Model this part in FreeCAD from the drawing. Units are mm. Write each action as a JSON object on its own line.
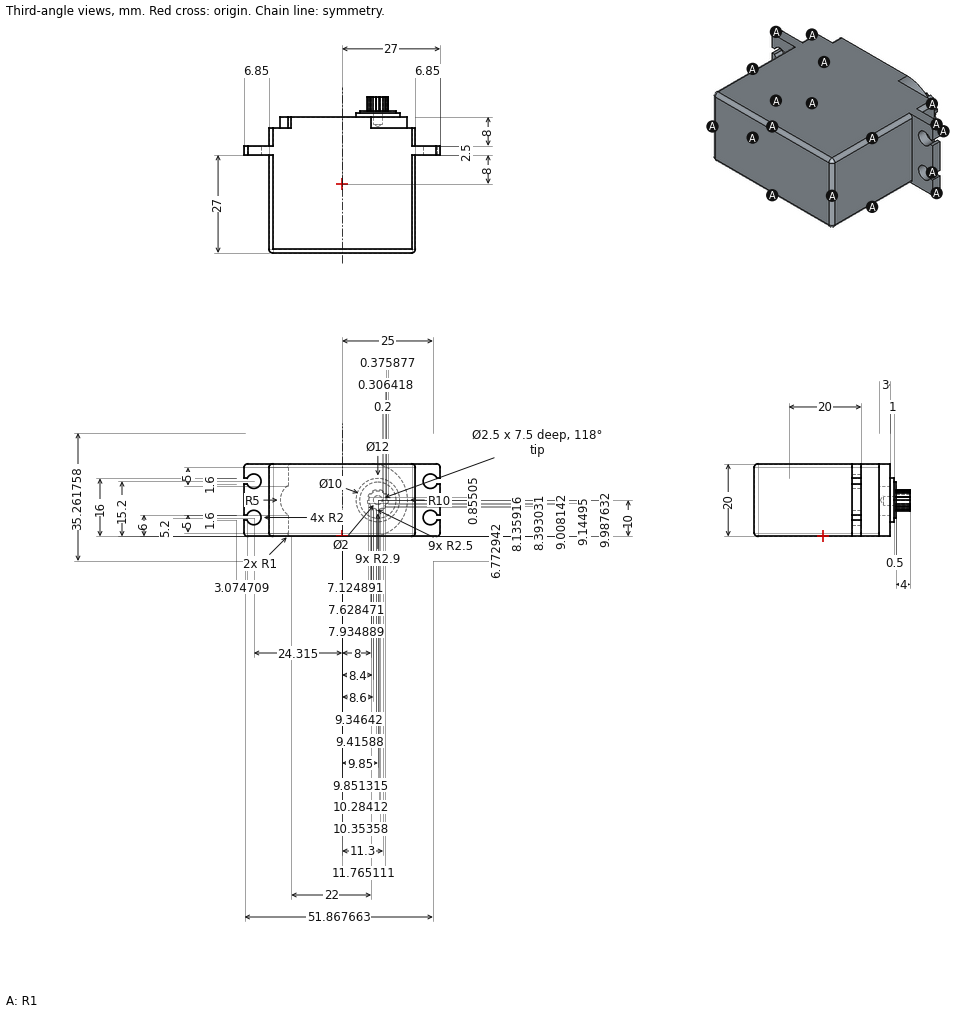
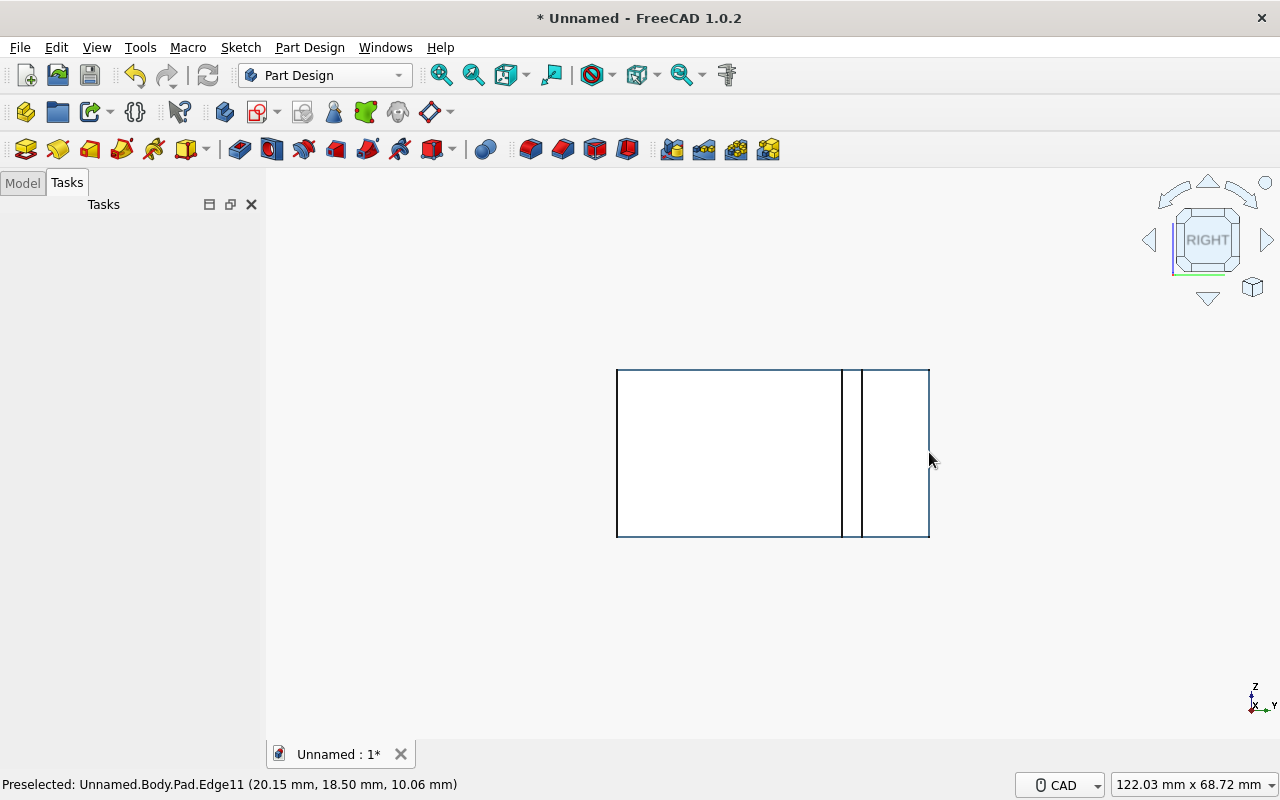
{"action": "key", "text": "5"}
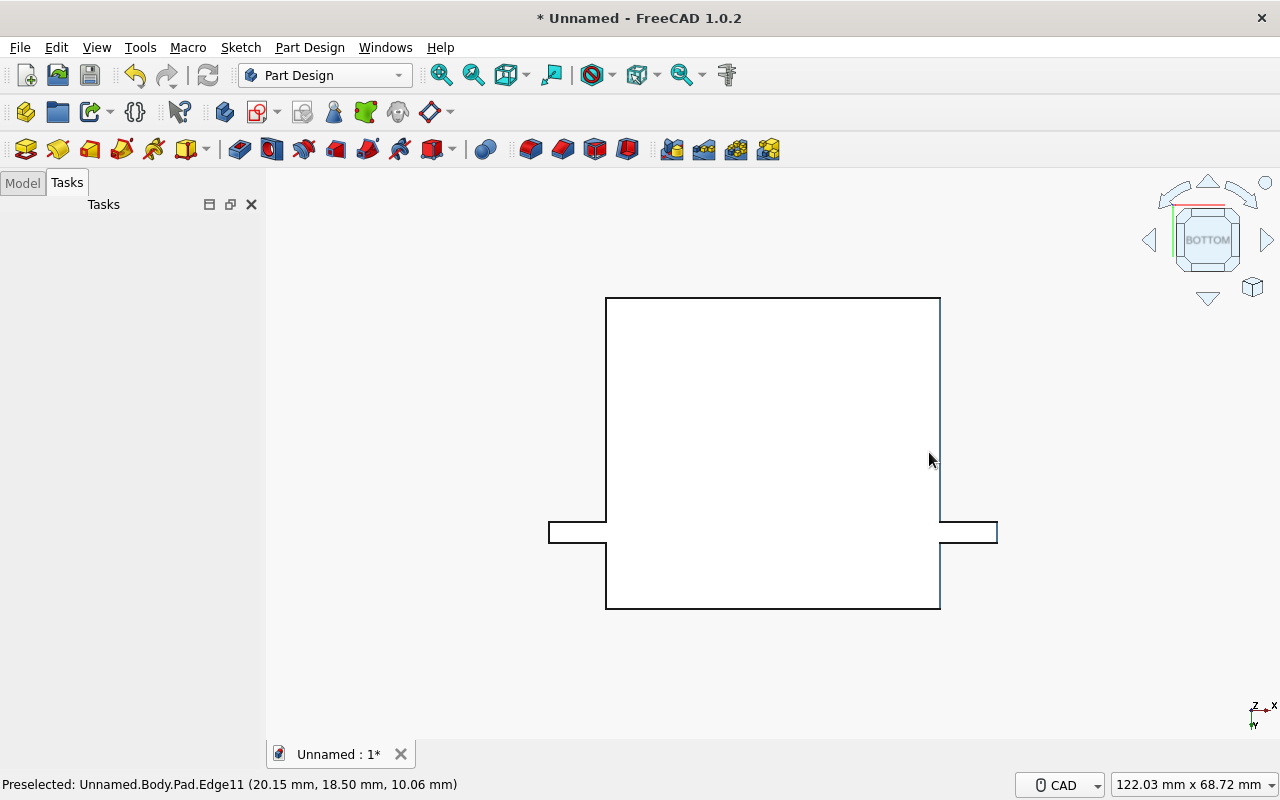
{"action": "left_click", "coordinate": [606, 409], "text": "ctrl"}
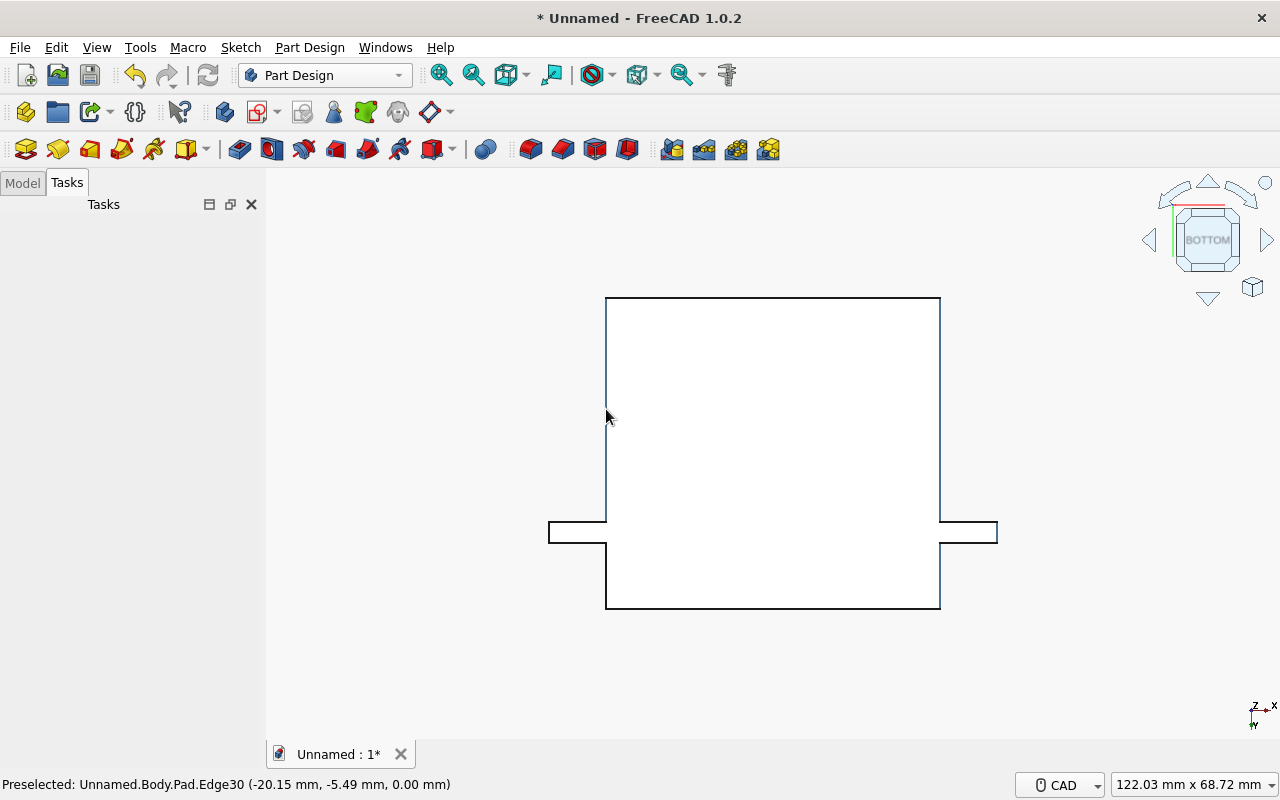
{"action": "left_click", "coordinate": [549, 531], "text": "ctrl"}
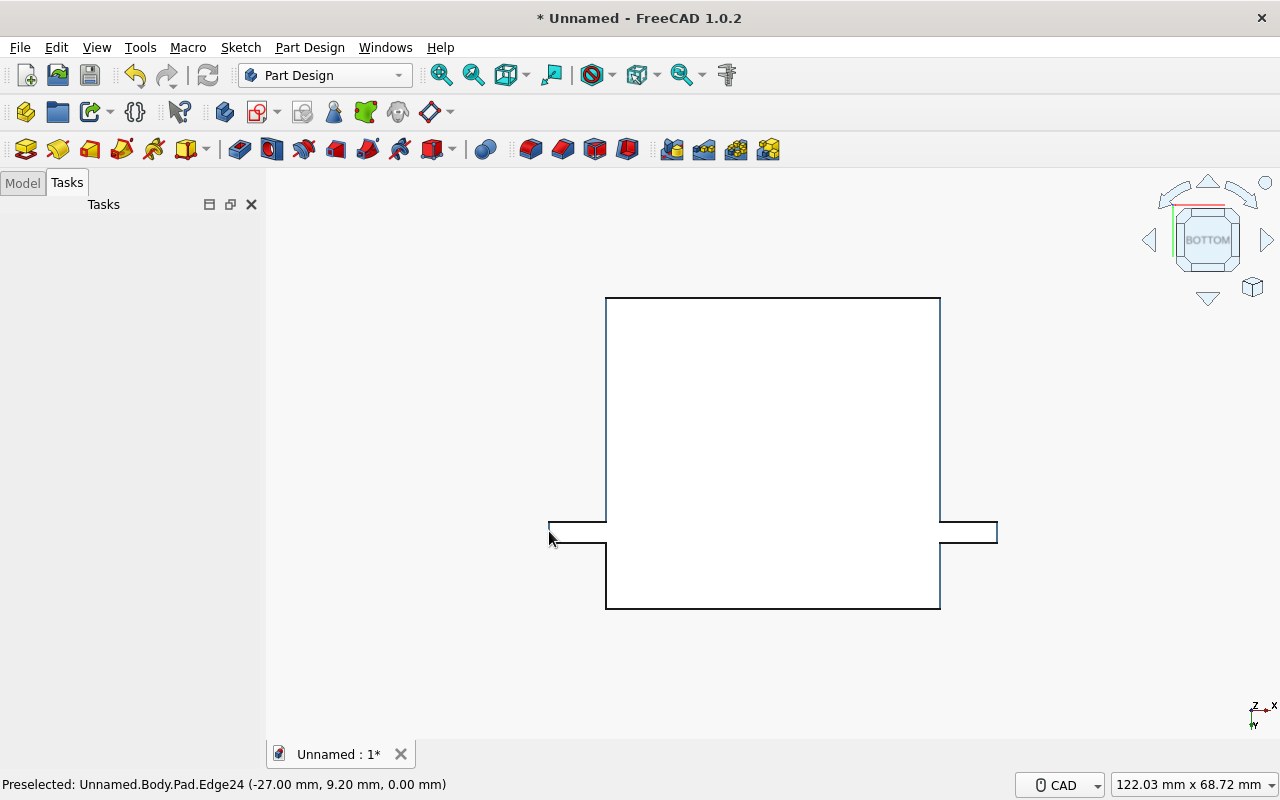
{"action": "left_click", "coordinate": [606, 575], "text": "ctrl"}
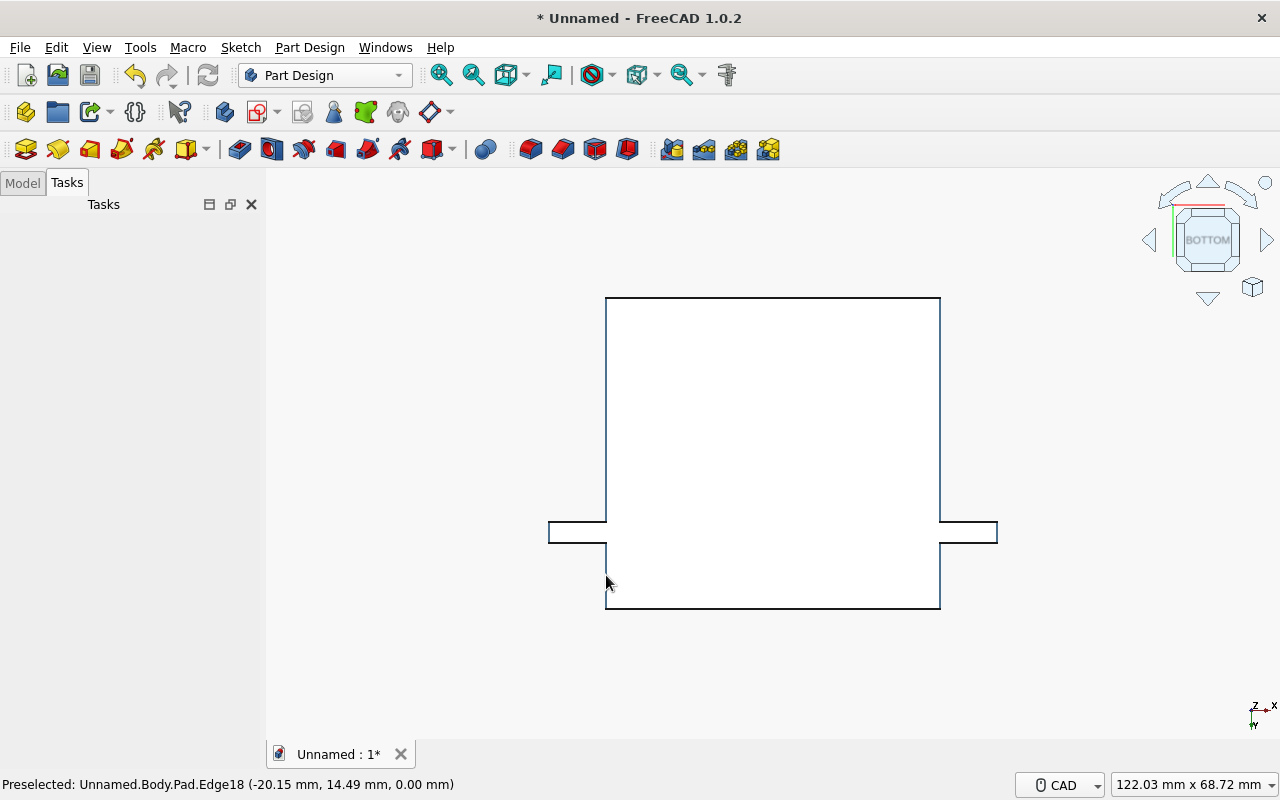
{"action": "key", "text": "4"}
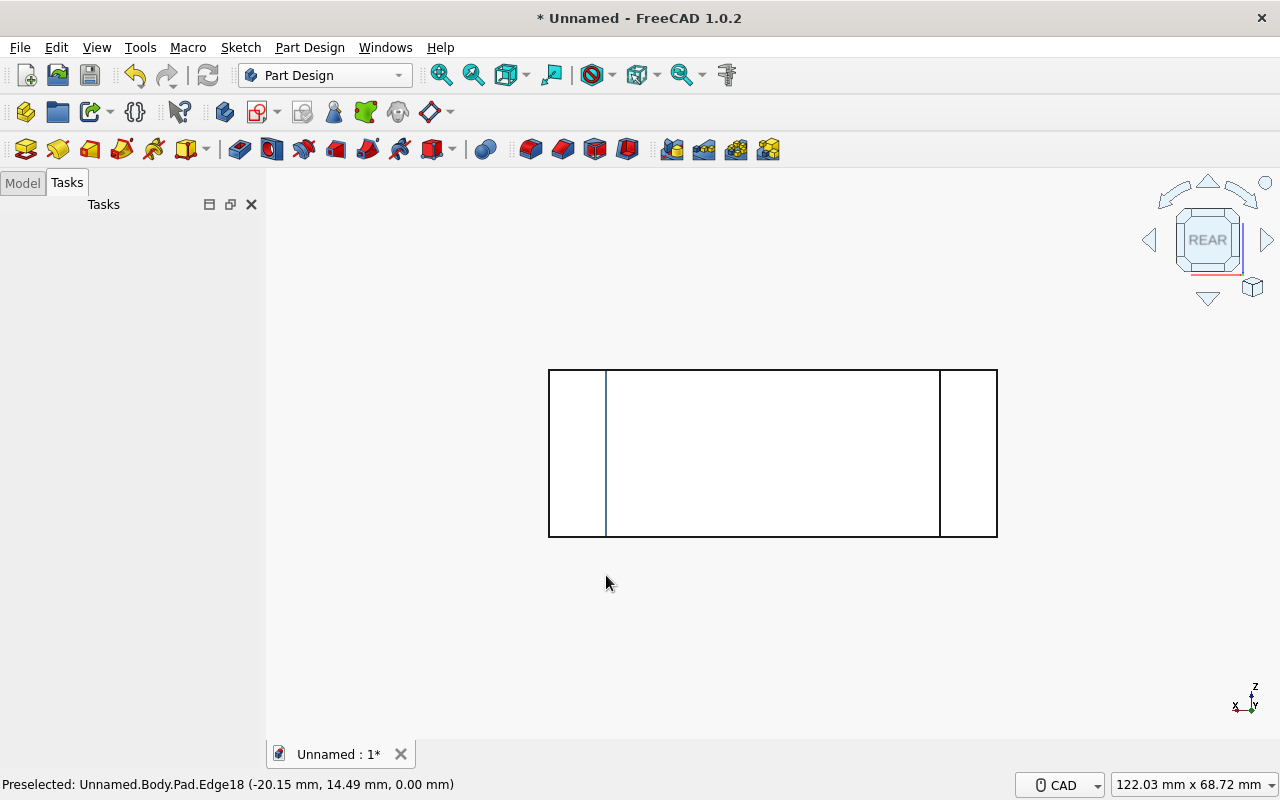
{"action": "left_click", "coordinate": [442, 76]}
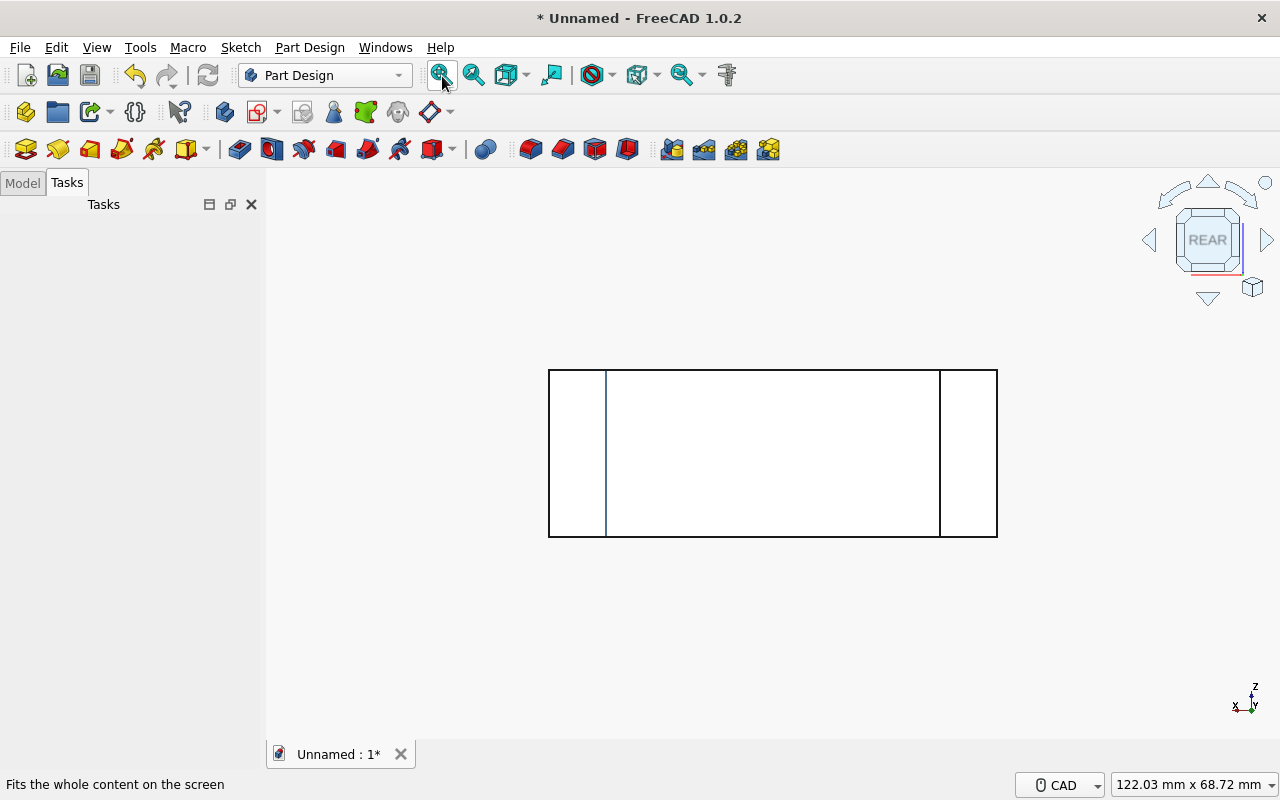
{"action": "left_click", "coordinate": [940, 453], "text": "ctrl"}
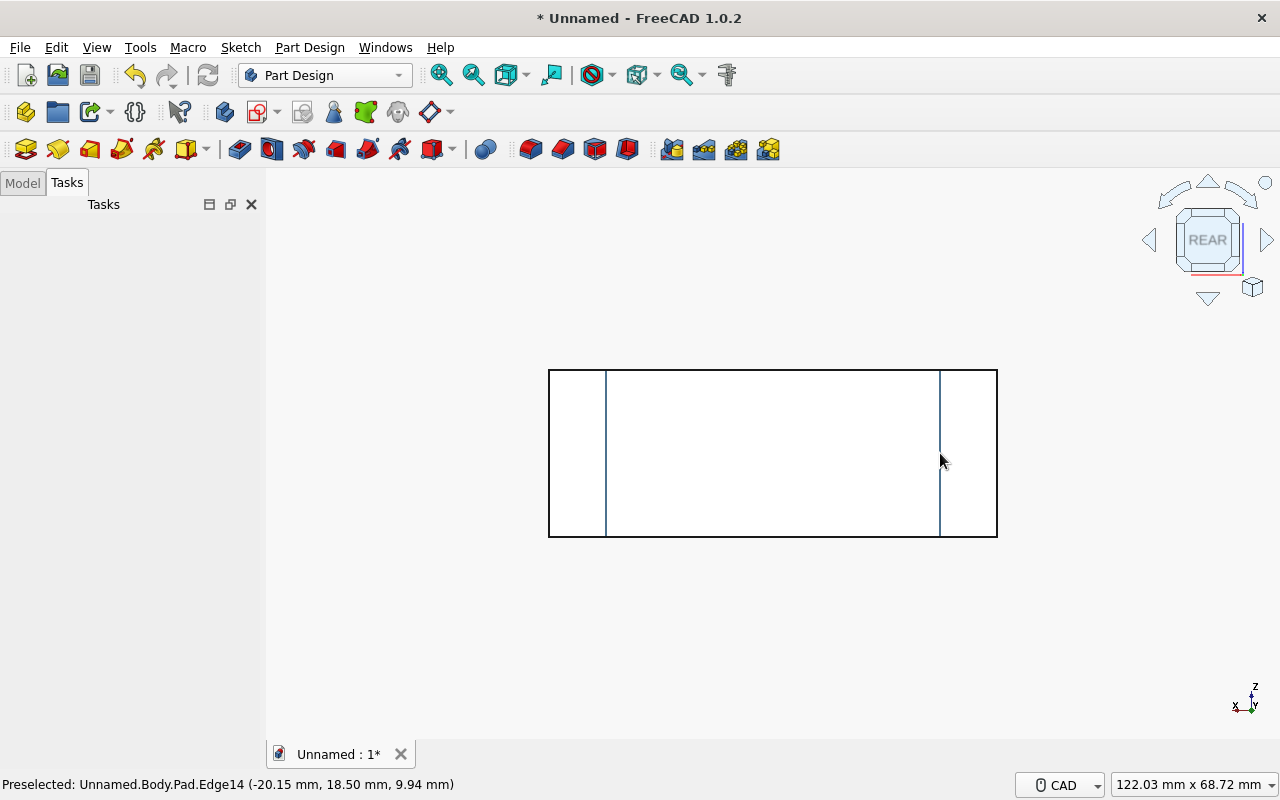
{"action": "left_click", "coordinate": [532, 150]}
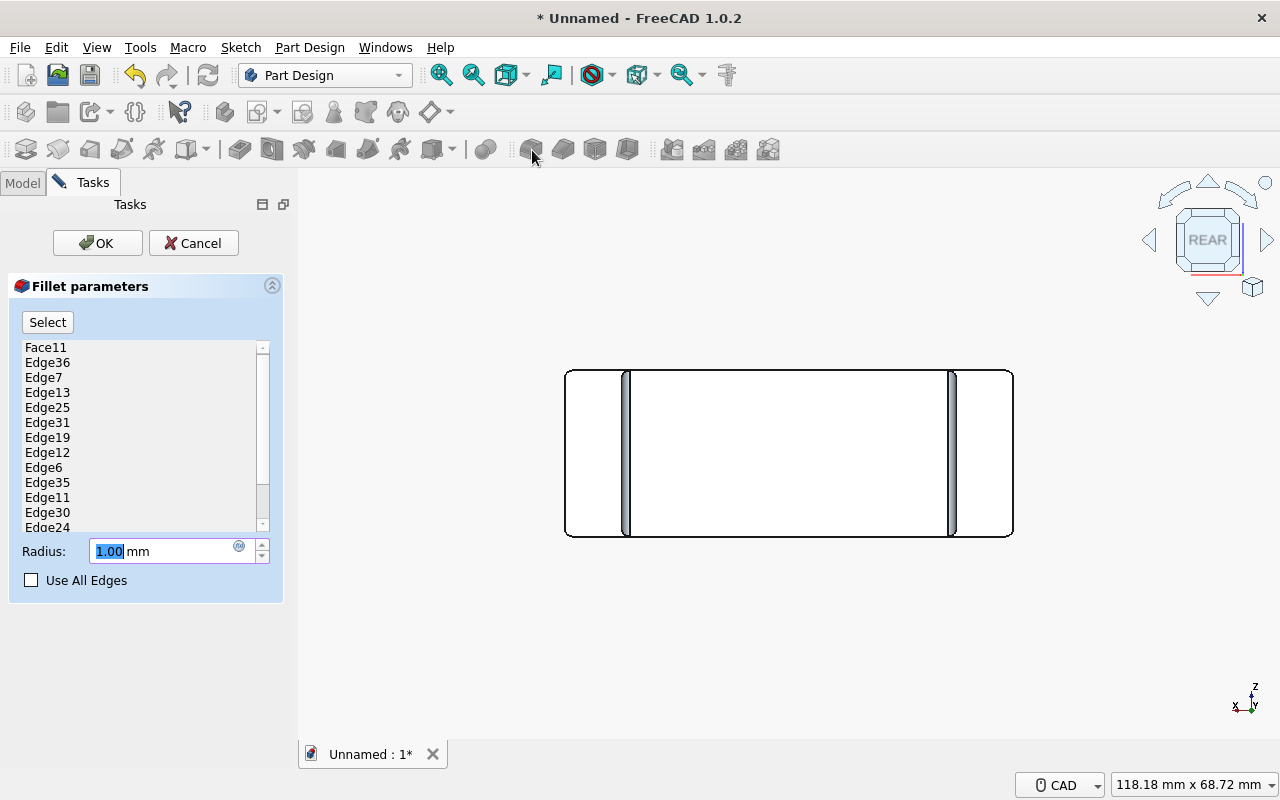
{"action": "type", "text": "1"}
{"action": "key", "text": "Tab"}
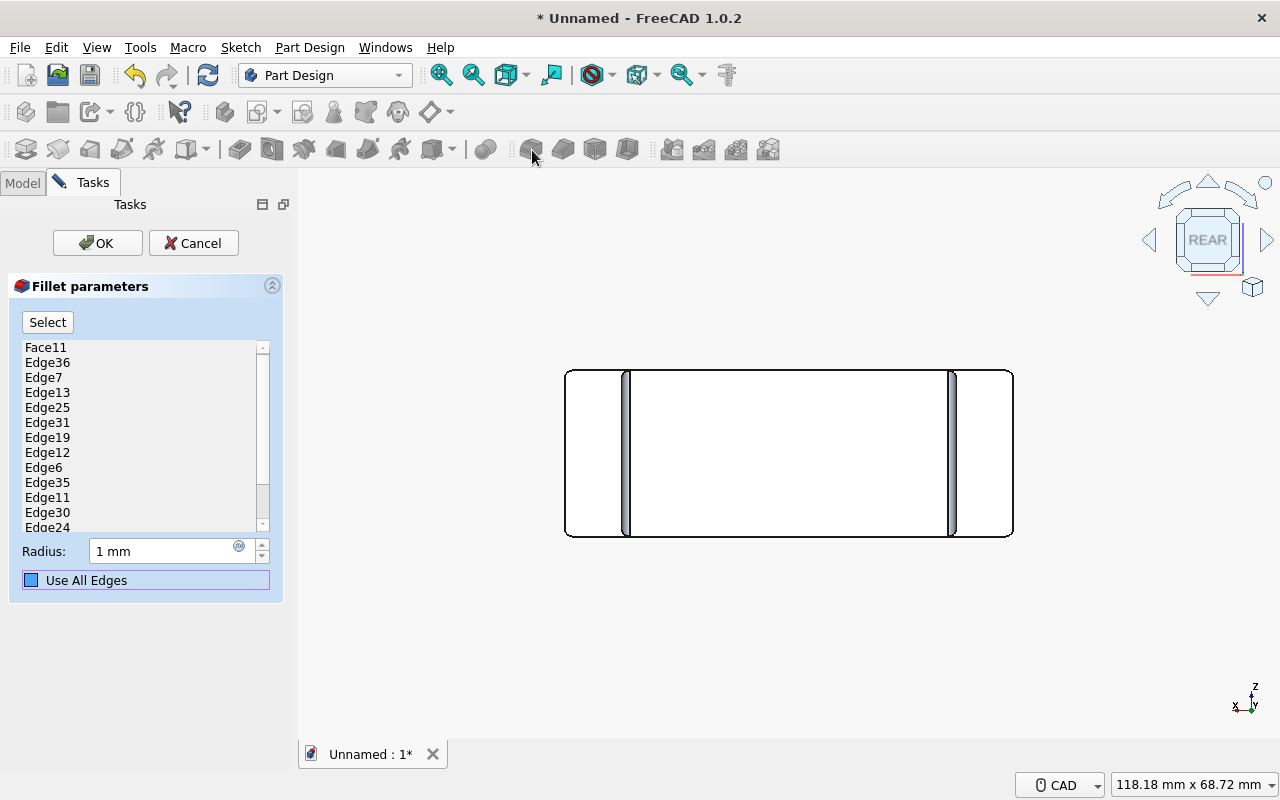
{"action": "left_click", "coordinate": [98, 243]}